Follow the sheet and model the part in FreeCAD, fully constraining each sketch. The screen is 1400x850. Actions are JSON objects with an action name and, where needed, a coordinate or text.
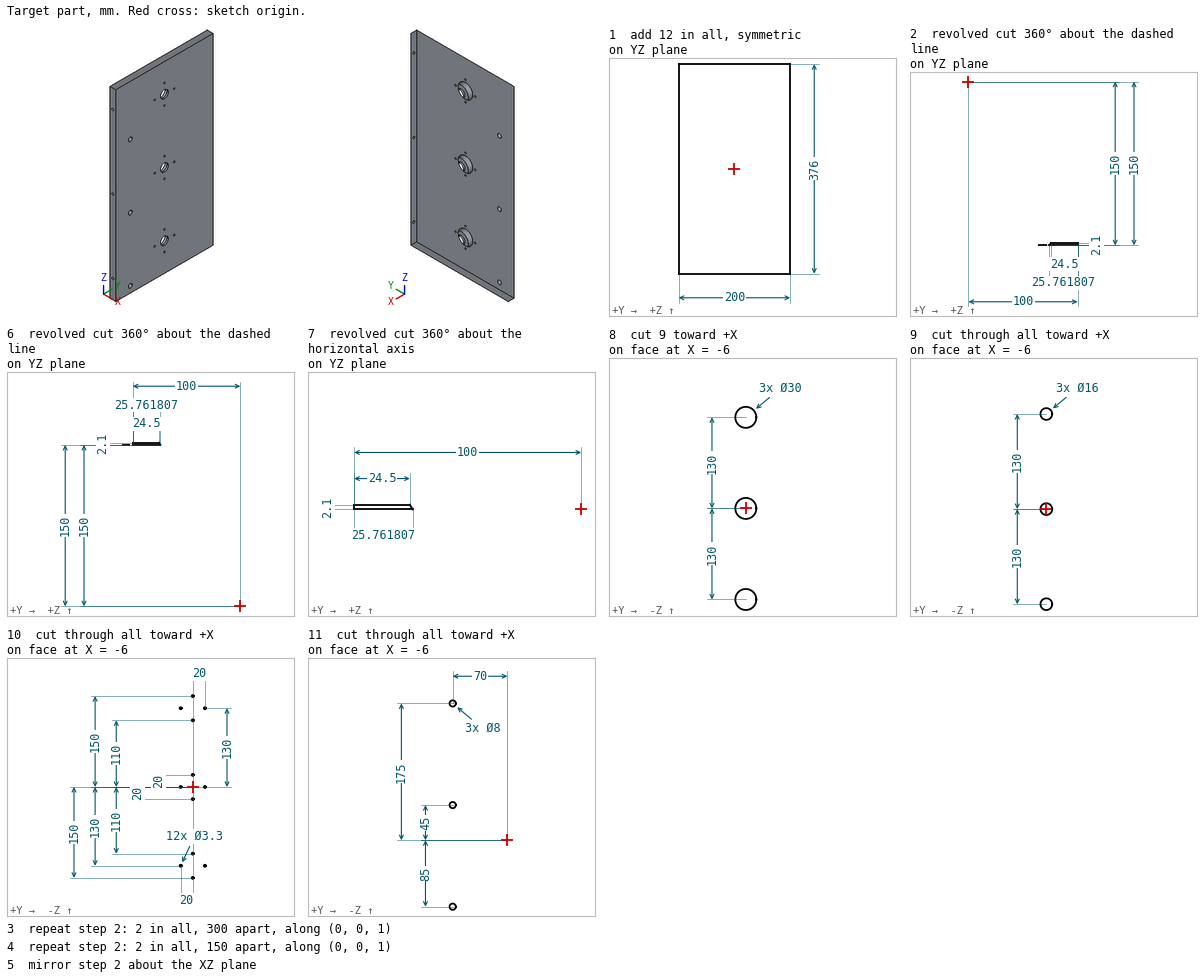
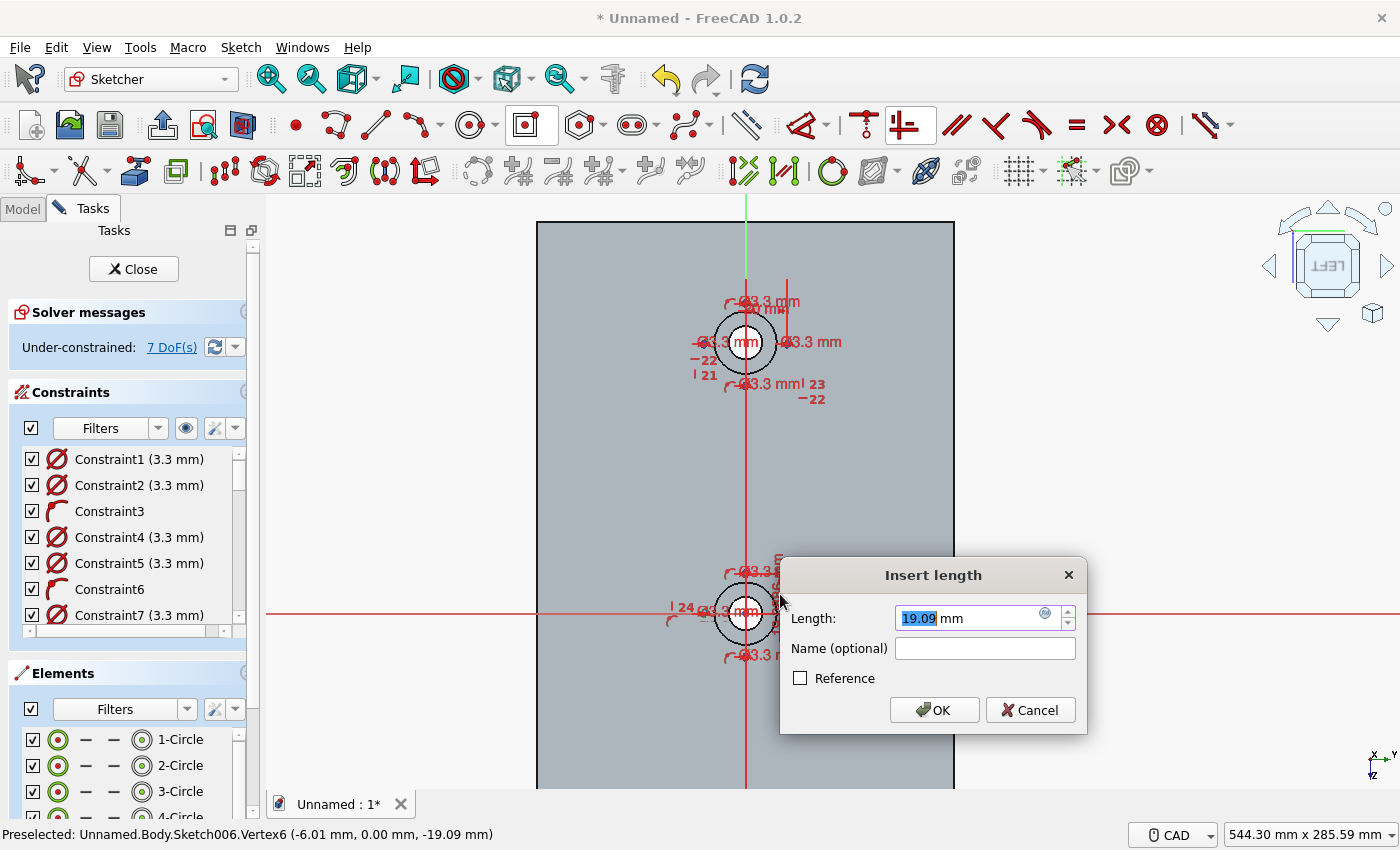
{"action": "type", "text": "20"}
{"action": "key", "text": "Return"}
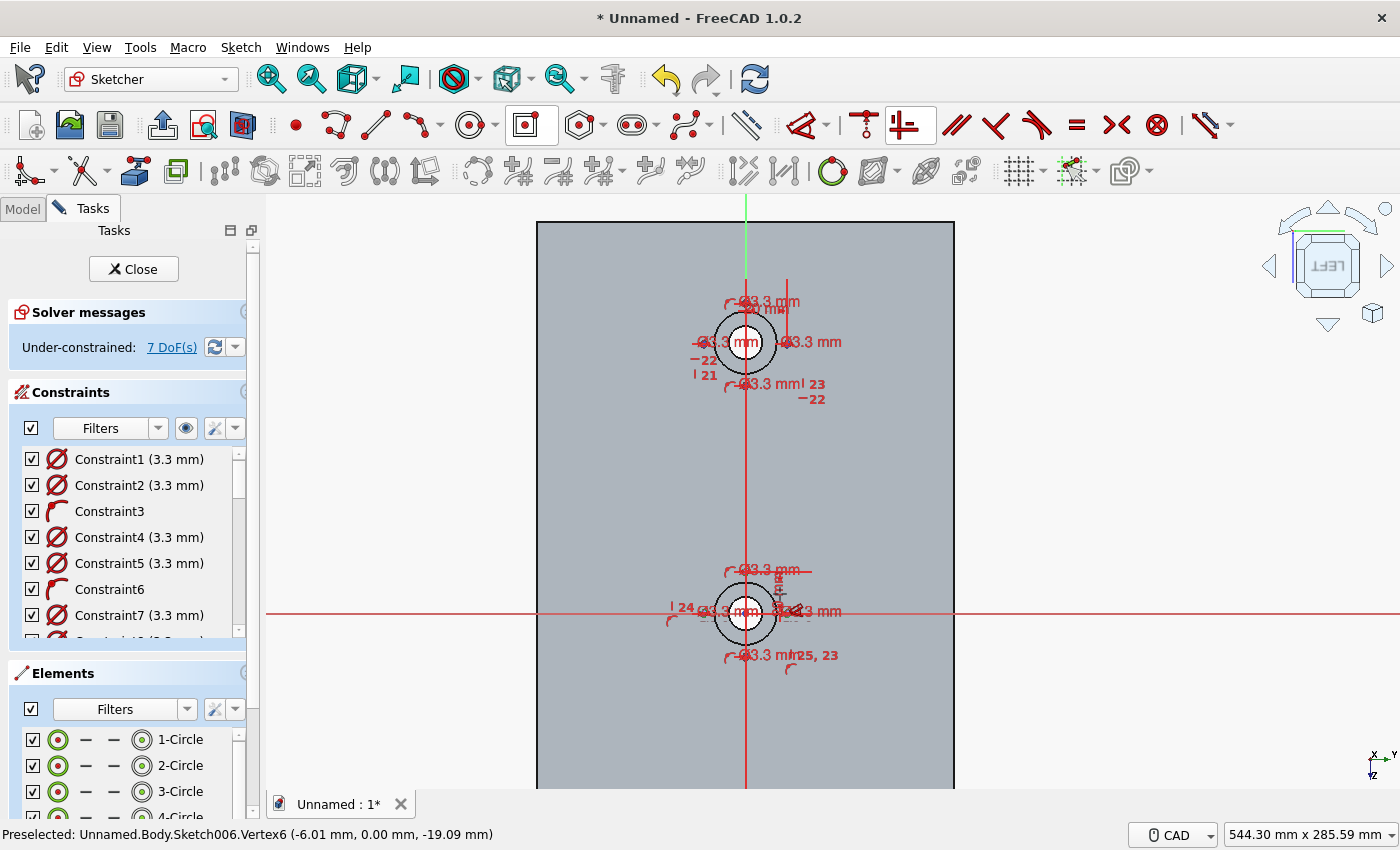
{"action": "left_click", "coordinate": [746, 657]}
{"action": "left_click", "coordinate": [780, 635]}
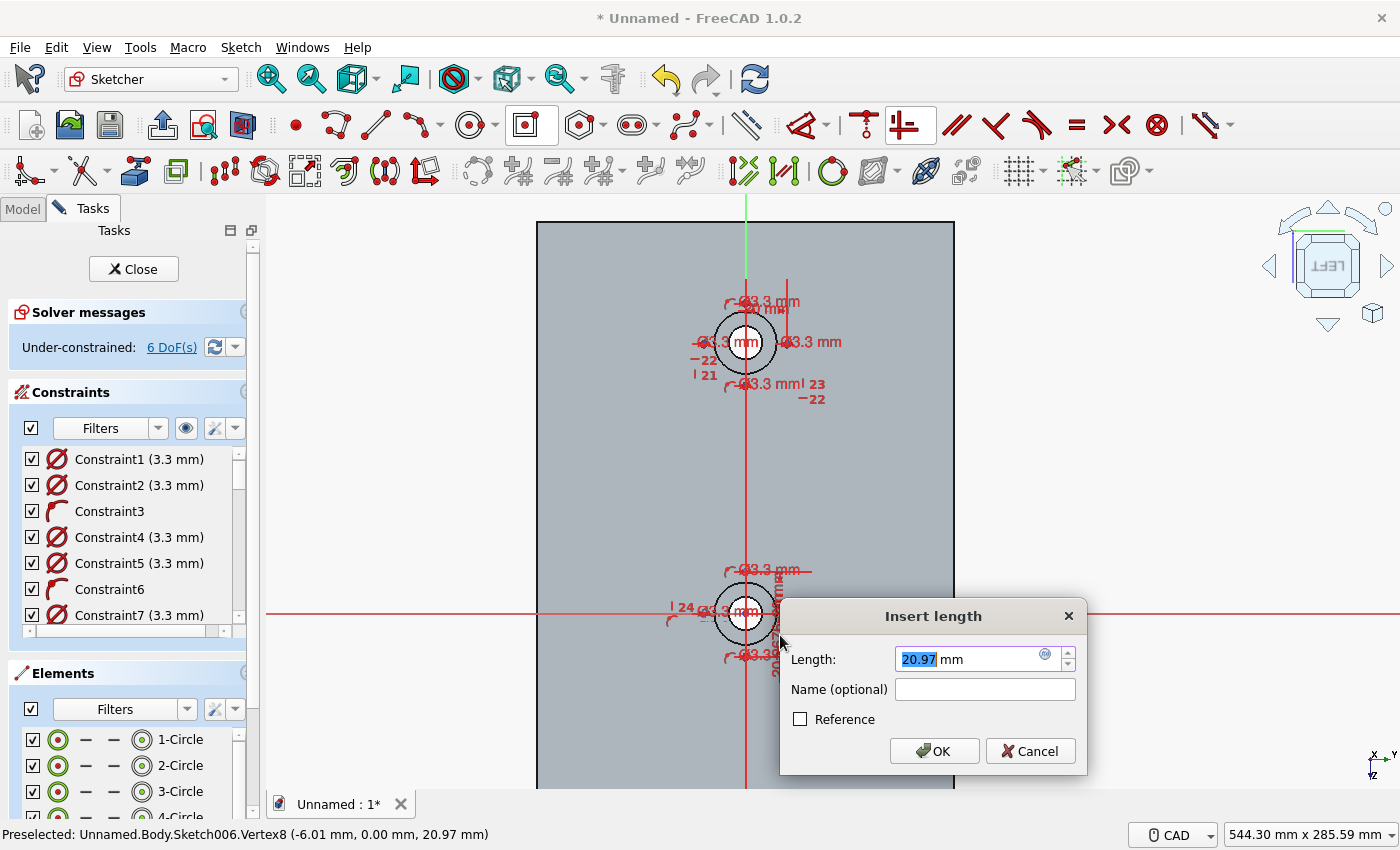
{"action": "type", "text": "20"}
{"action": "key", "text": "Return"}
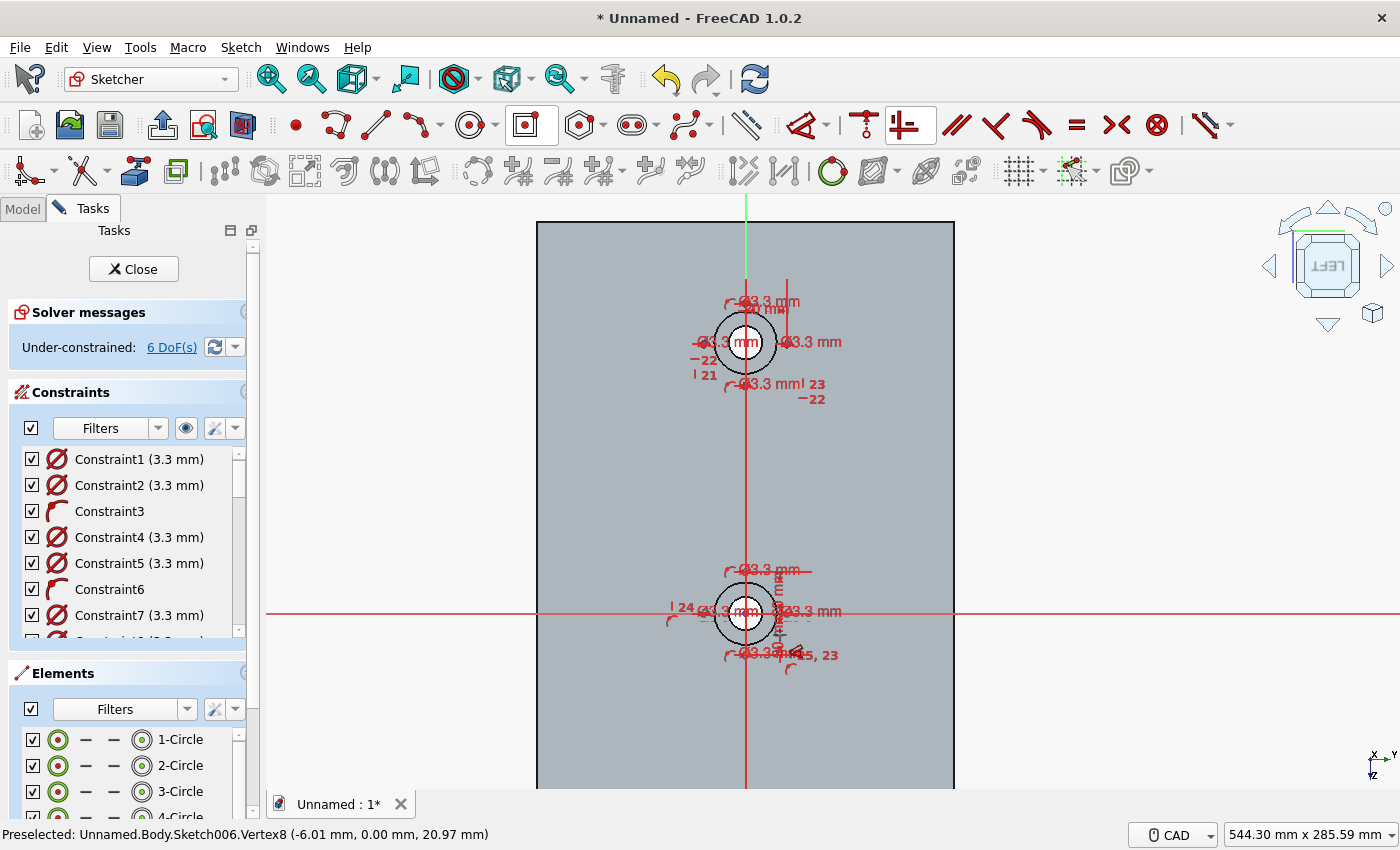
{"action": "scroll", "coordinate": [788, 343], "scroll_direction": "down", "scroll_amount": 3}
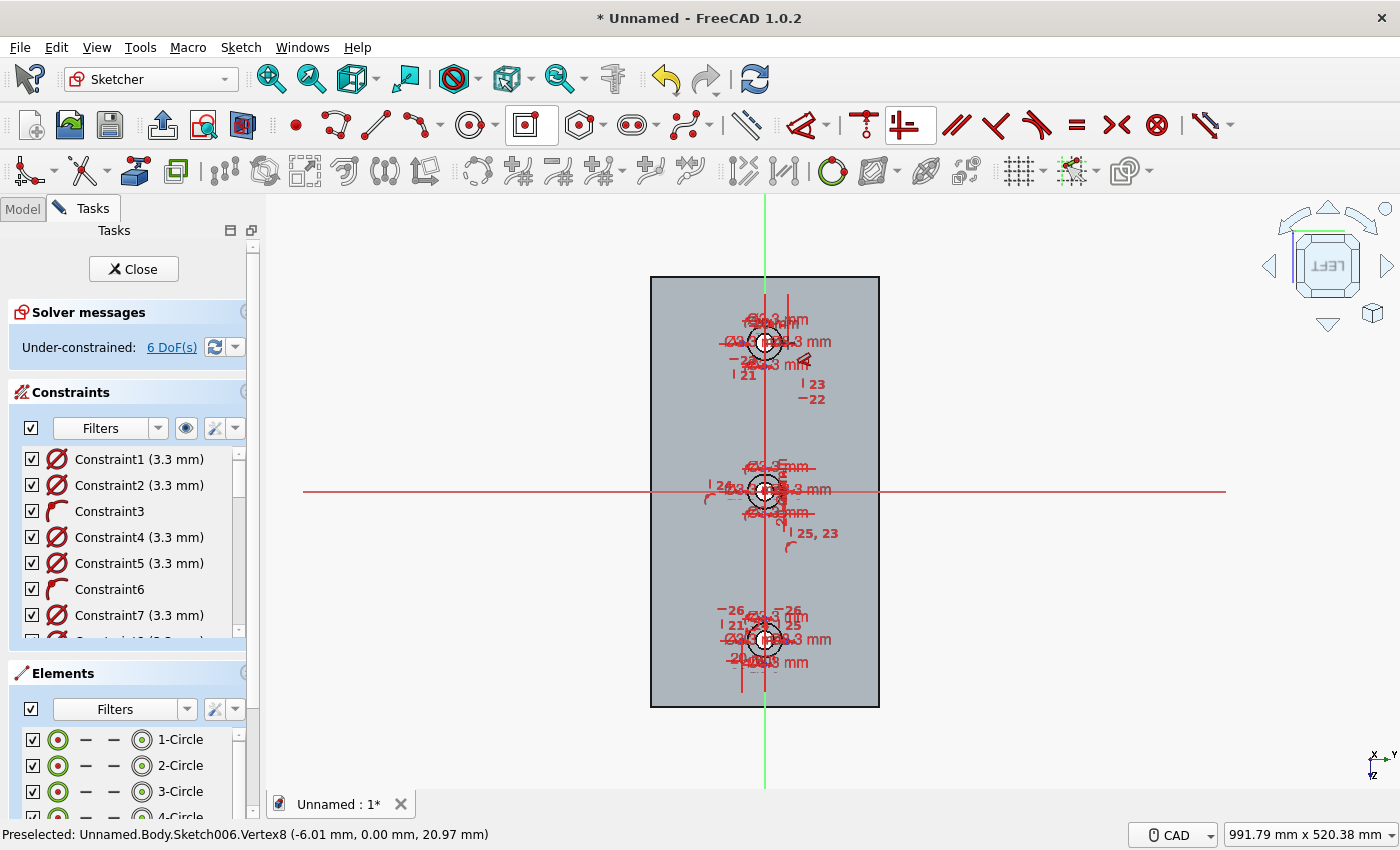
{"action": "left_click", "coordinate": [742, 641]}
{"action": "left_click", "coordinate": [708, 567]}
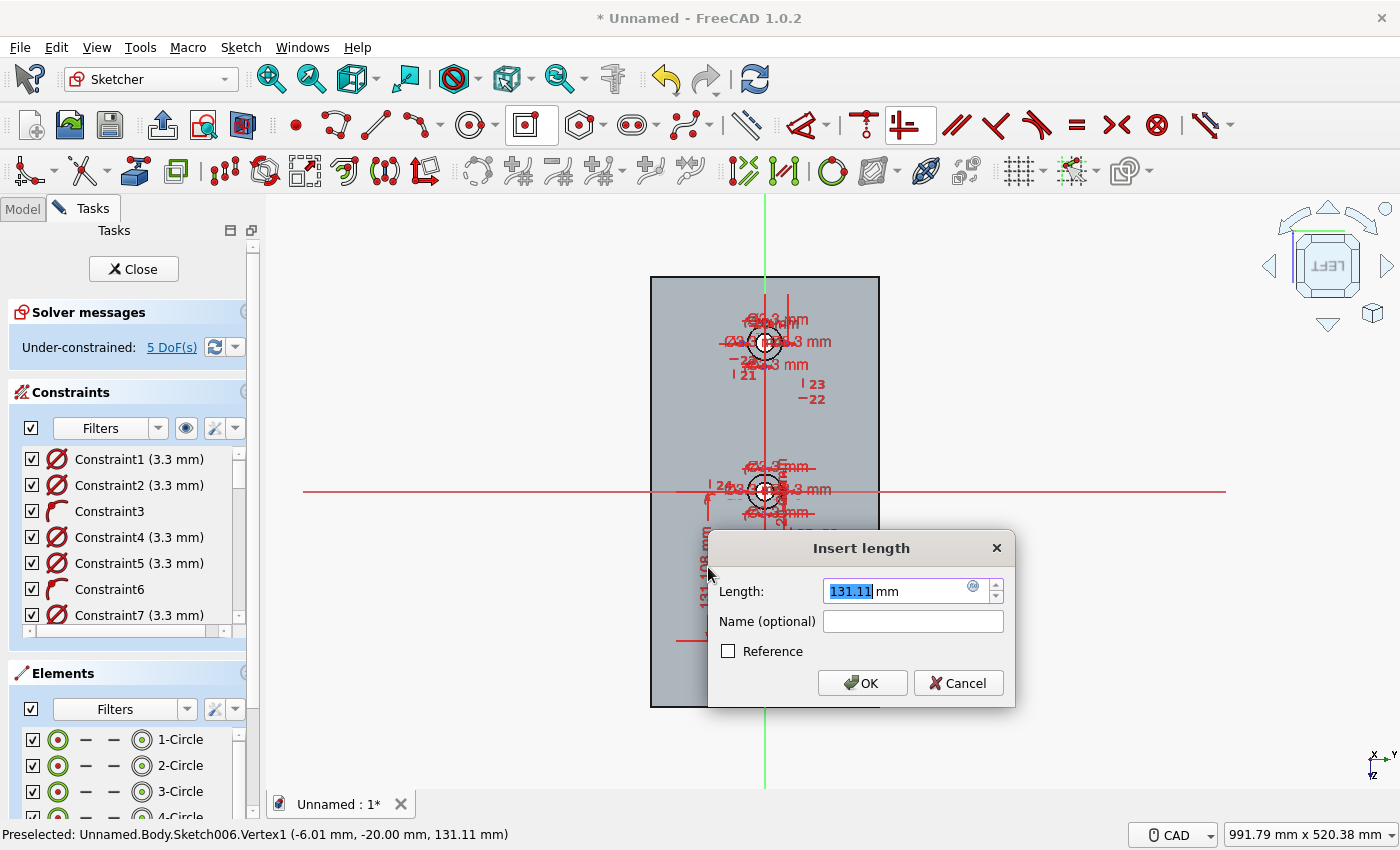
{"action": "type", "text": "130"}
{"action": "key", "text": "Return"}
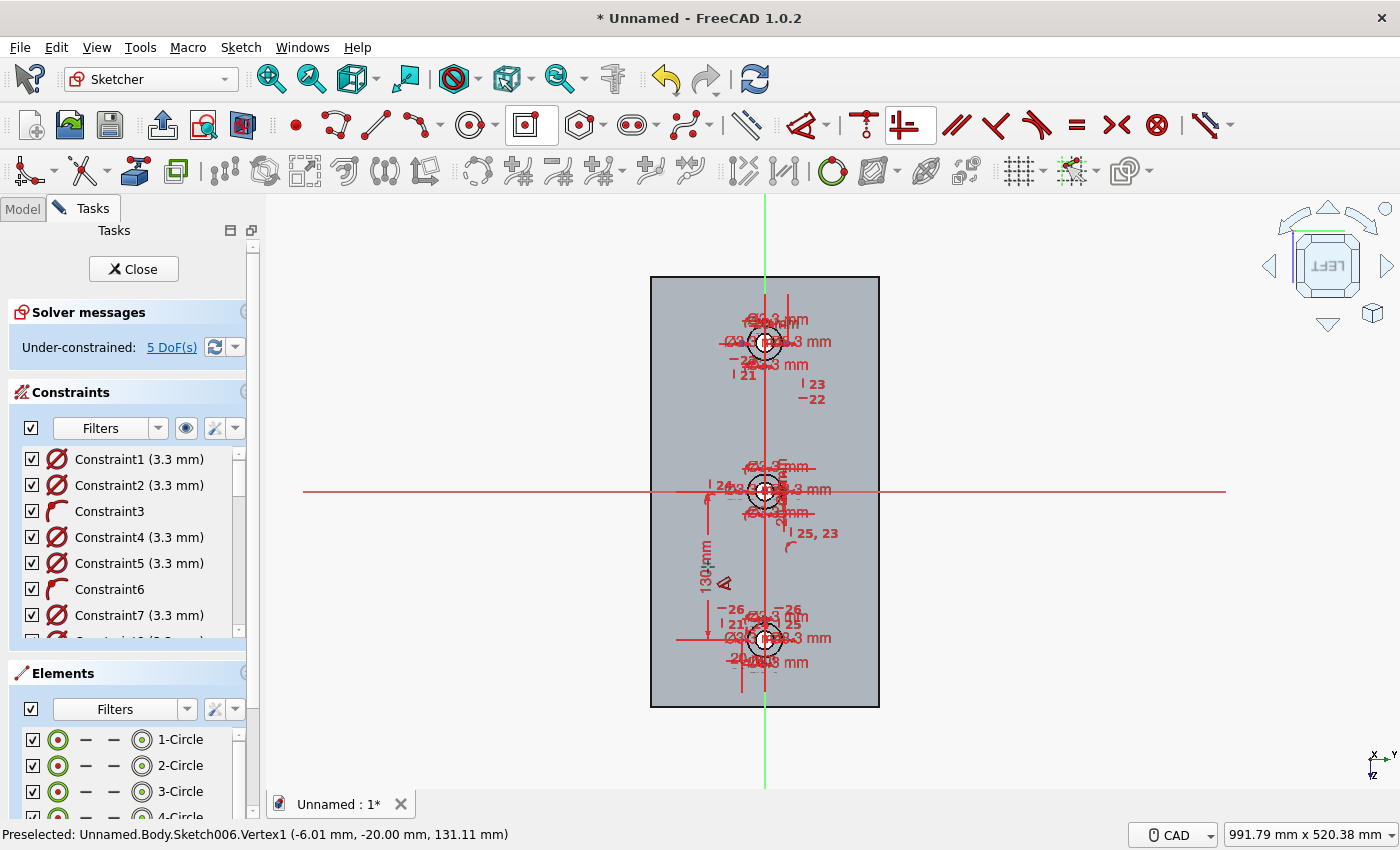
{"action": "left_click", "coordinate": [765, 321]}
{"action": "left_click", "coordinate": [799, 407]}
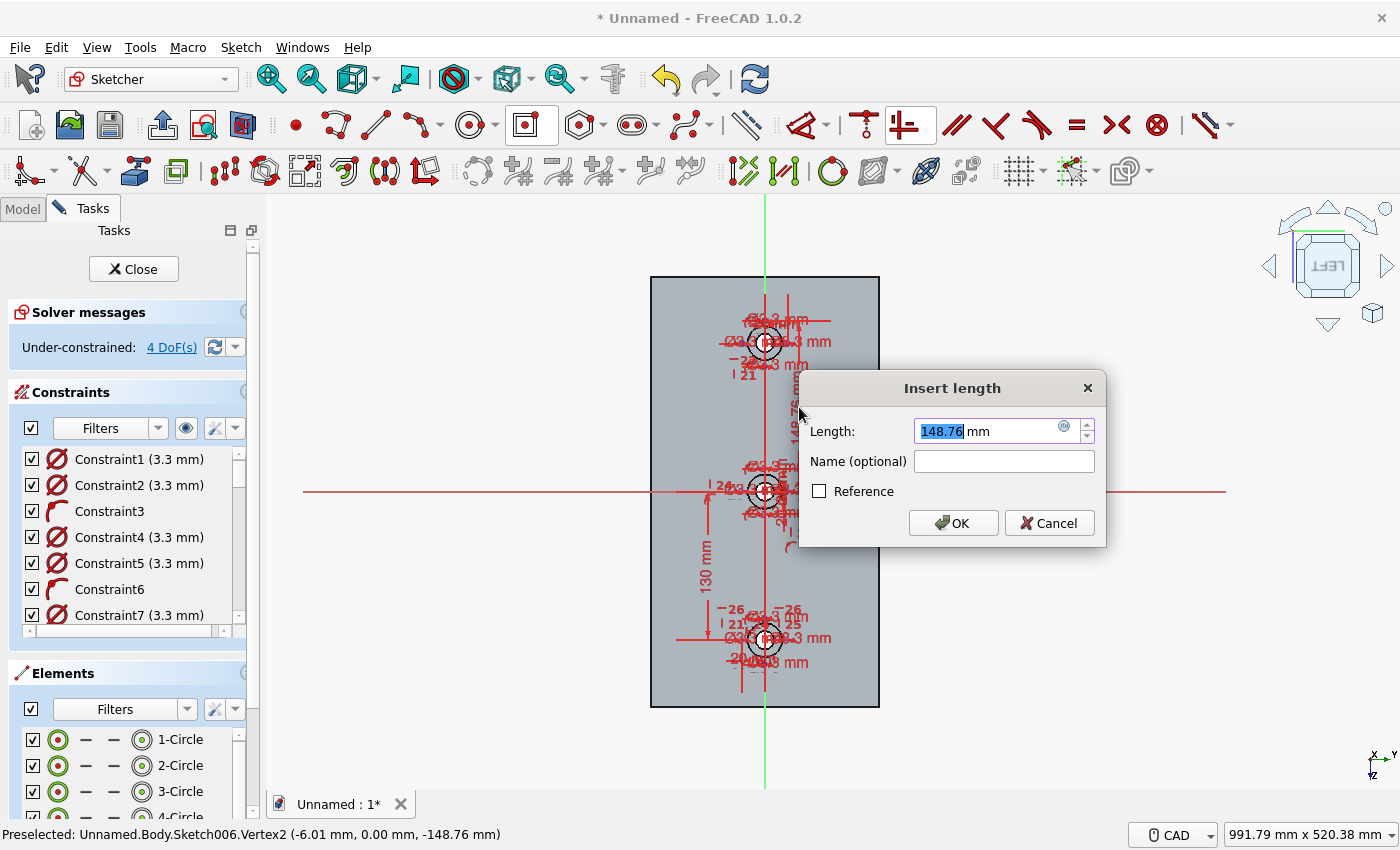
{"action": "type", "text": "150"}
{"action": "key", "text": "Return"}